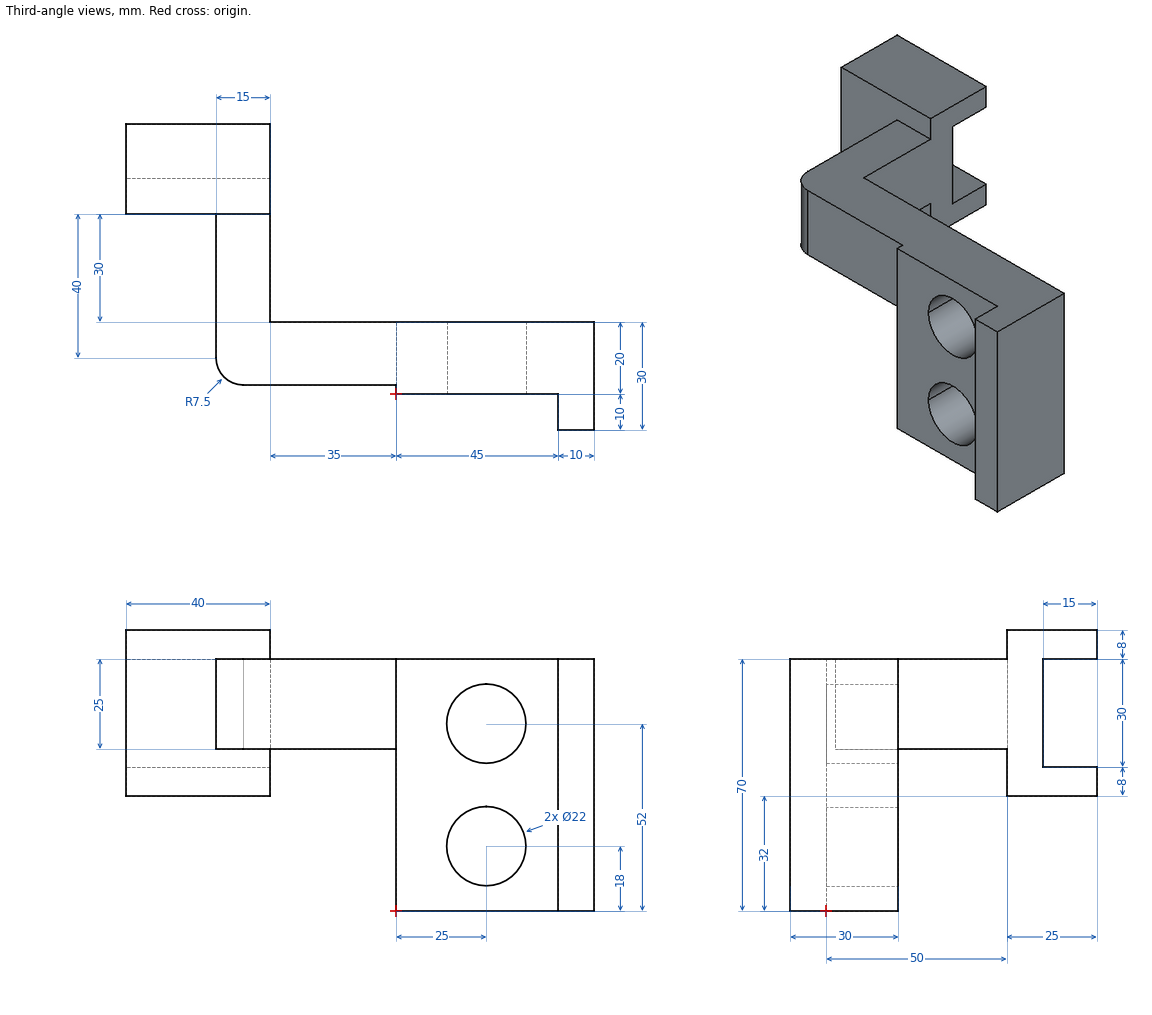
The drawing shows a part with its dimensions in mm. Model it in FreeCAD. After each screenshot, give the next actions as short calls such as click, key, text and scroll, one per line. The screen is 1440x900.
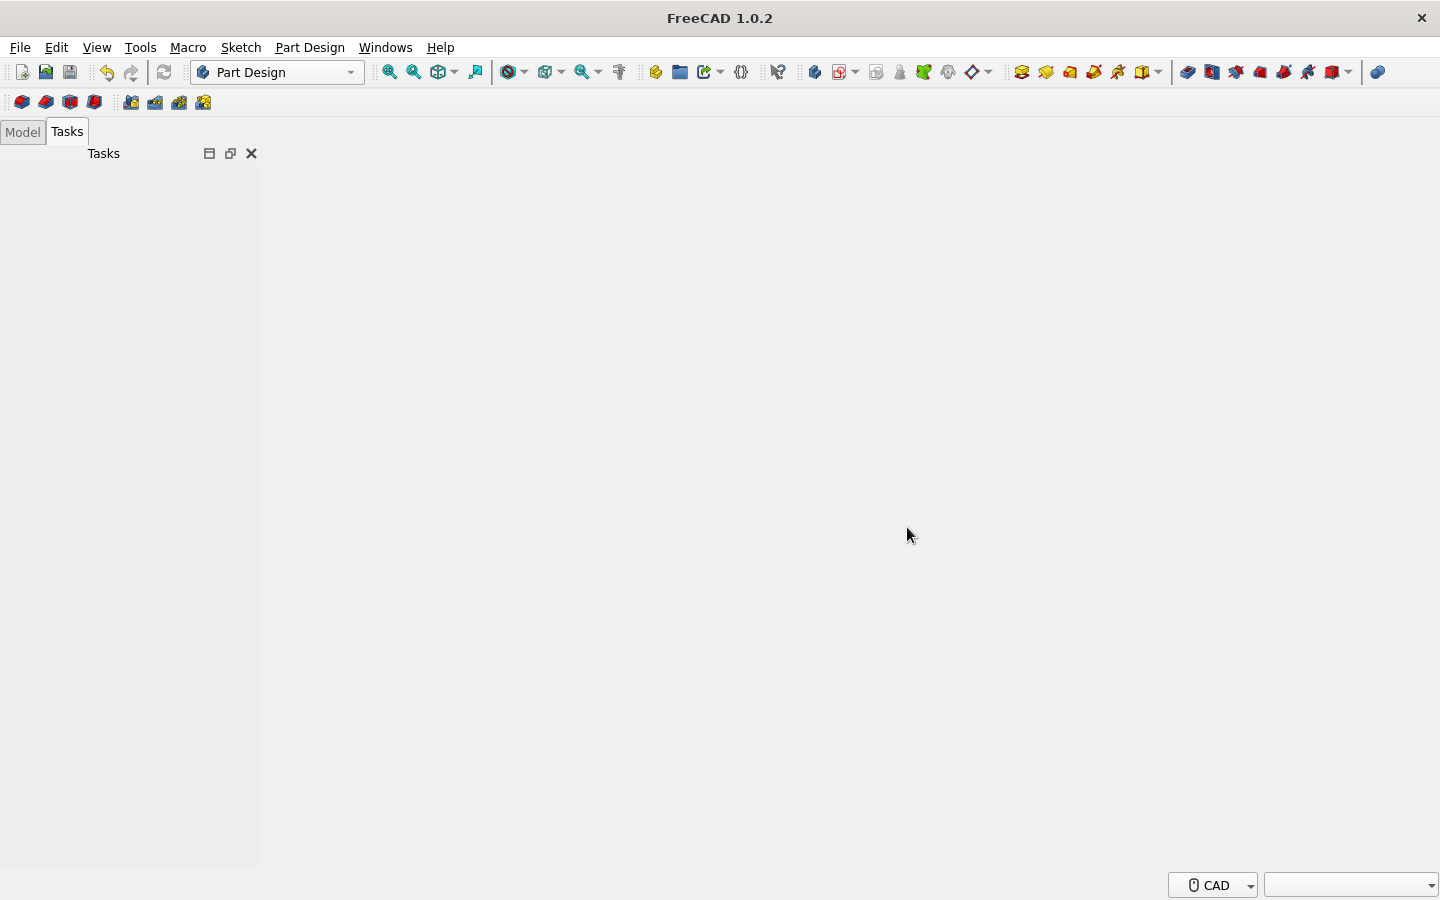
click(22, 72)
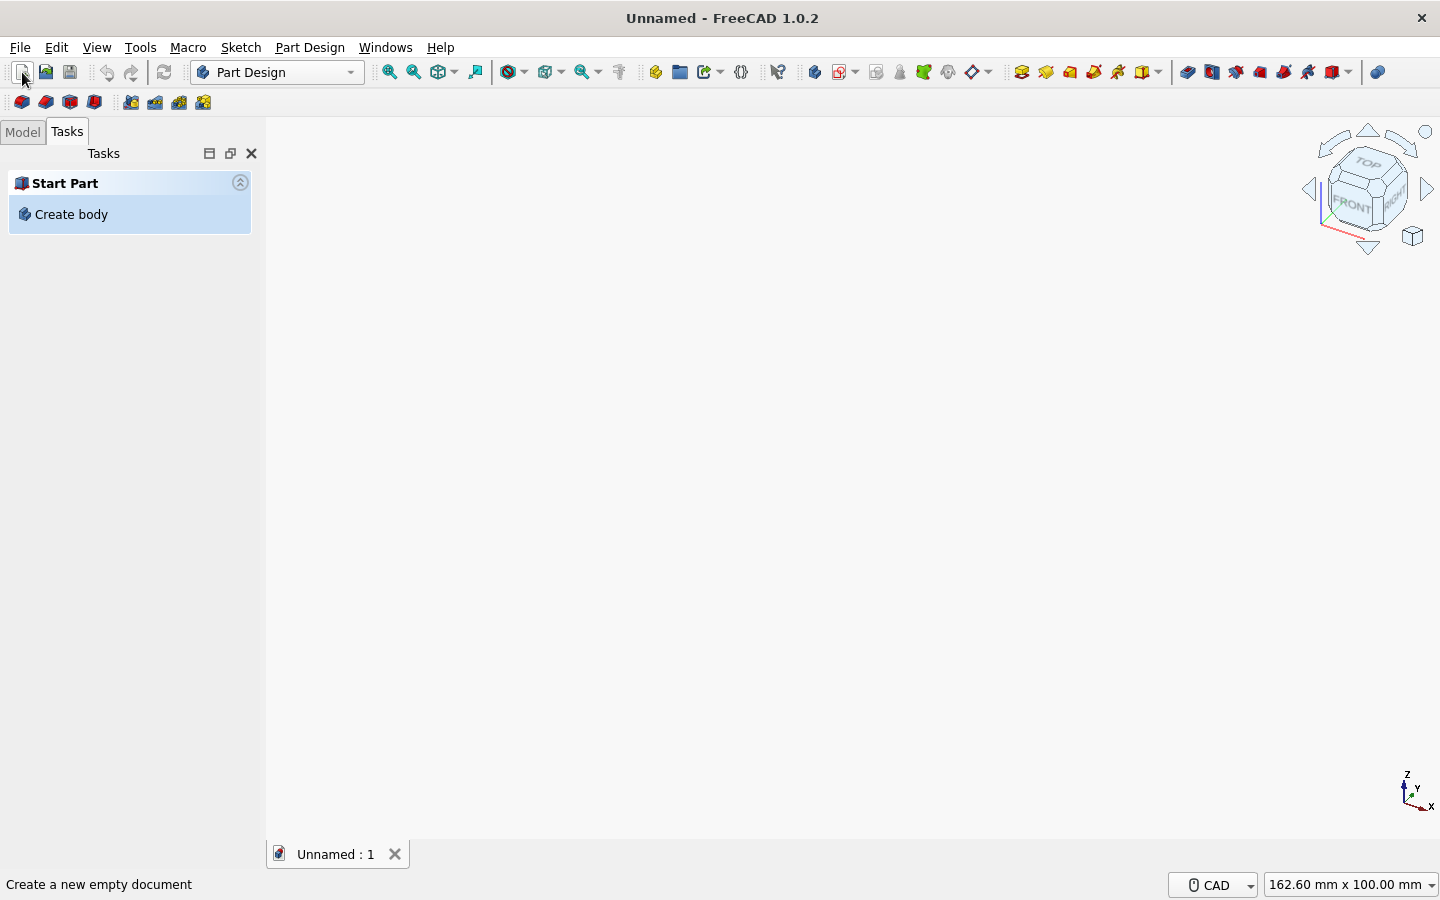
click(840, 72)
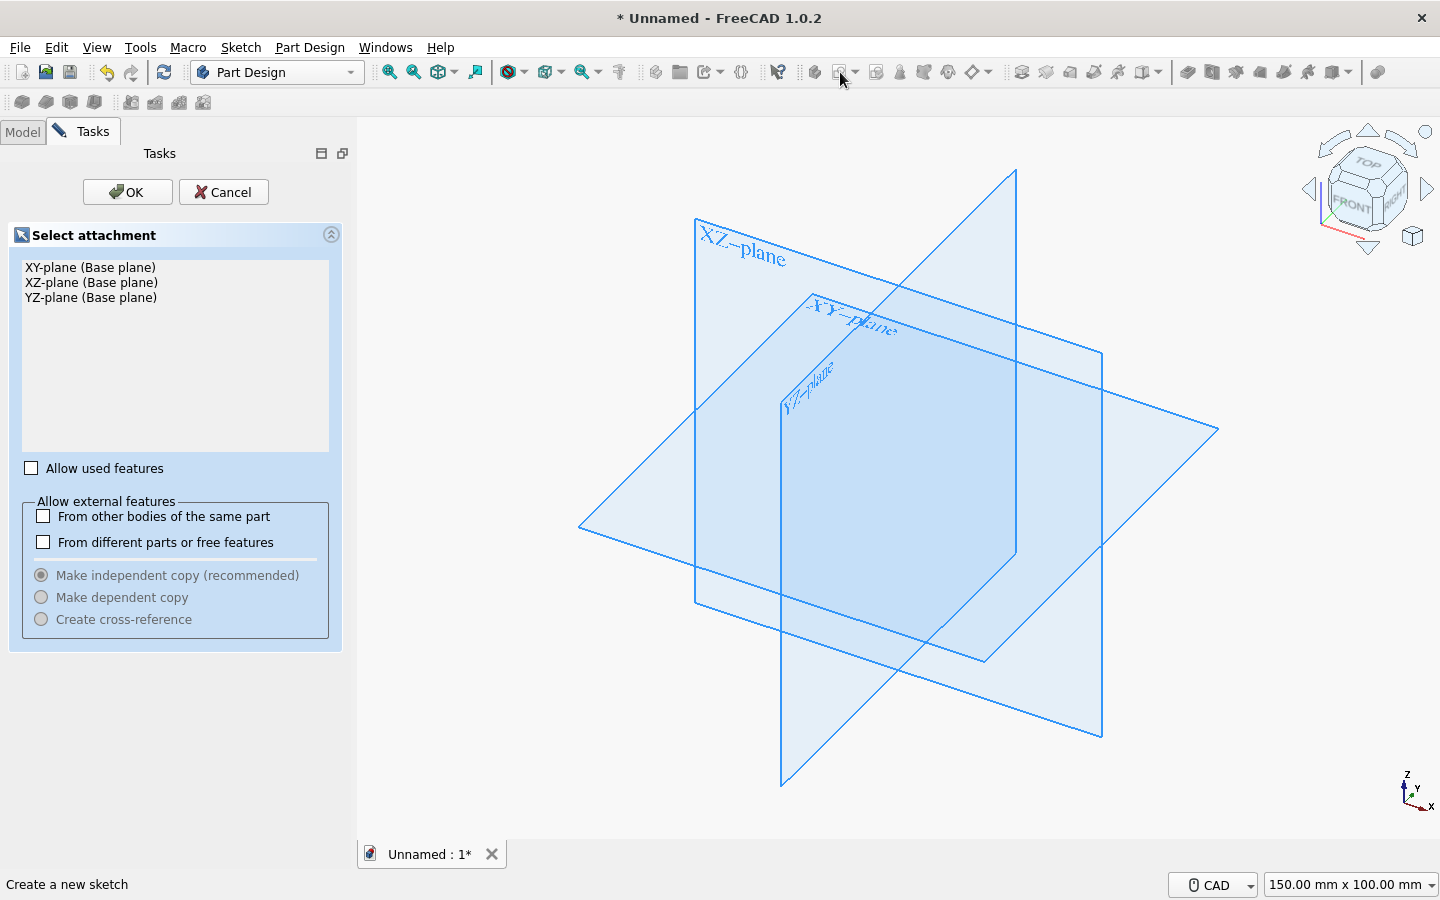
click(82, 268)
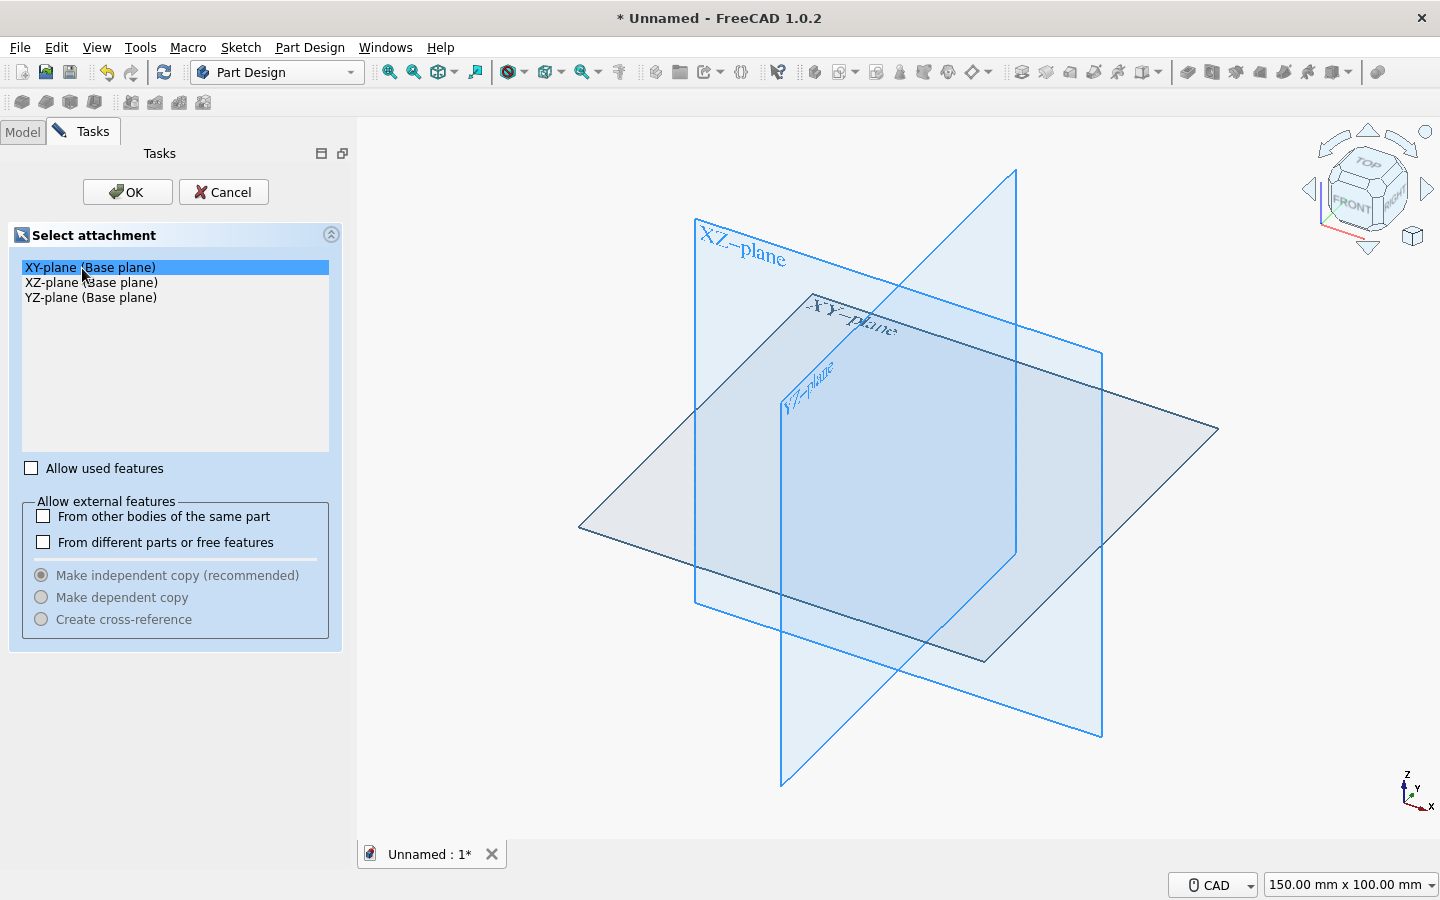
click(128, 192)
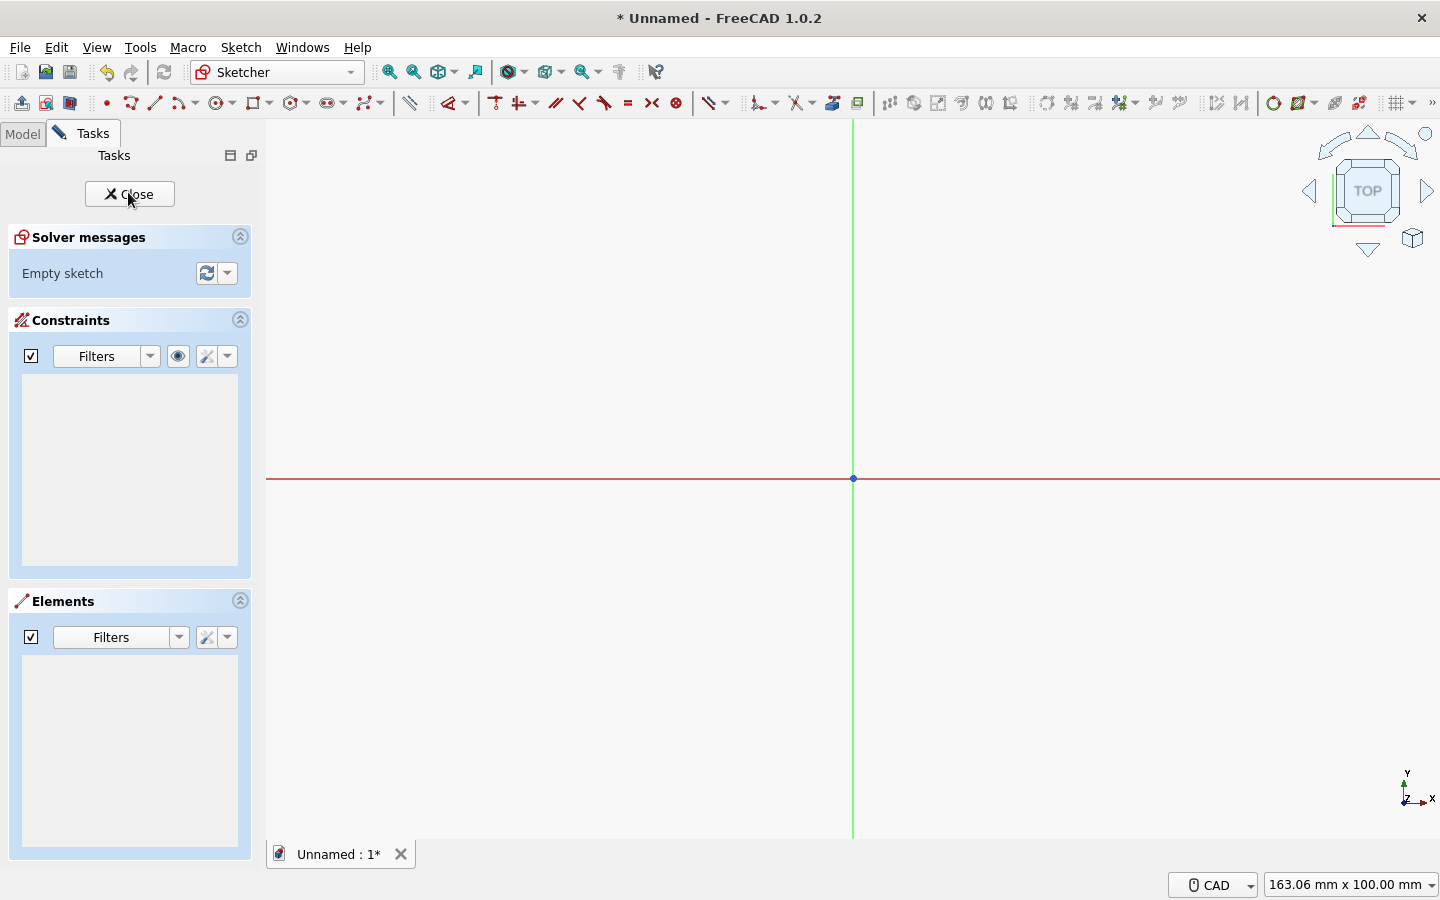
scroll(1275, 399, up, 3)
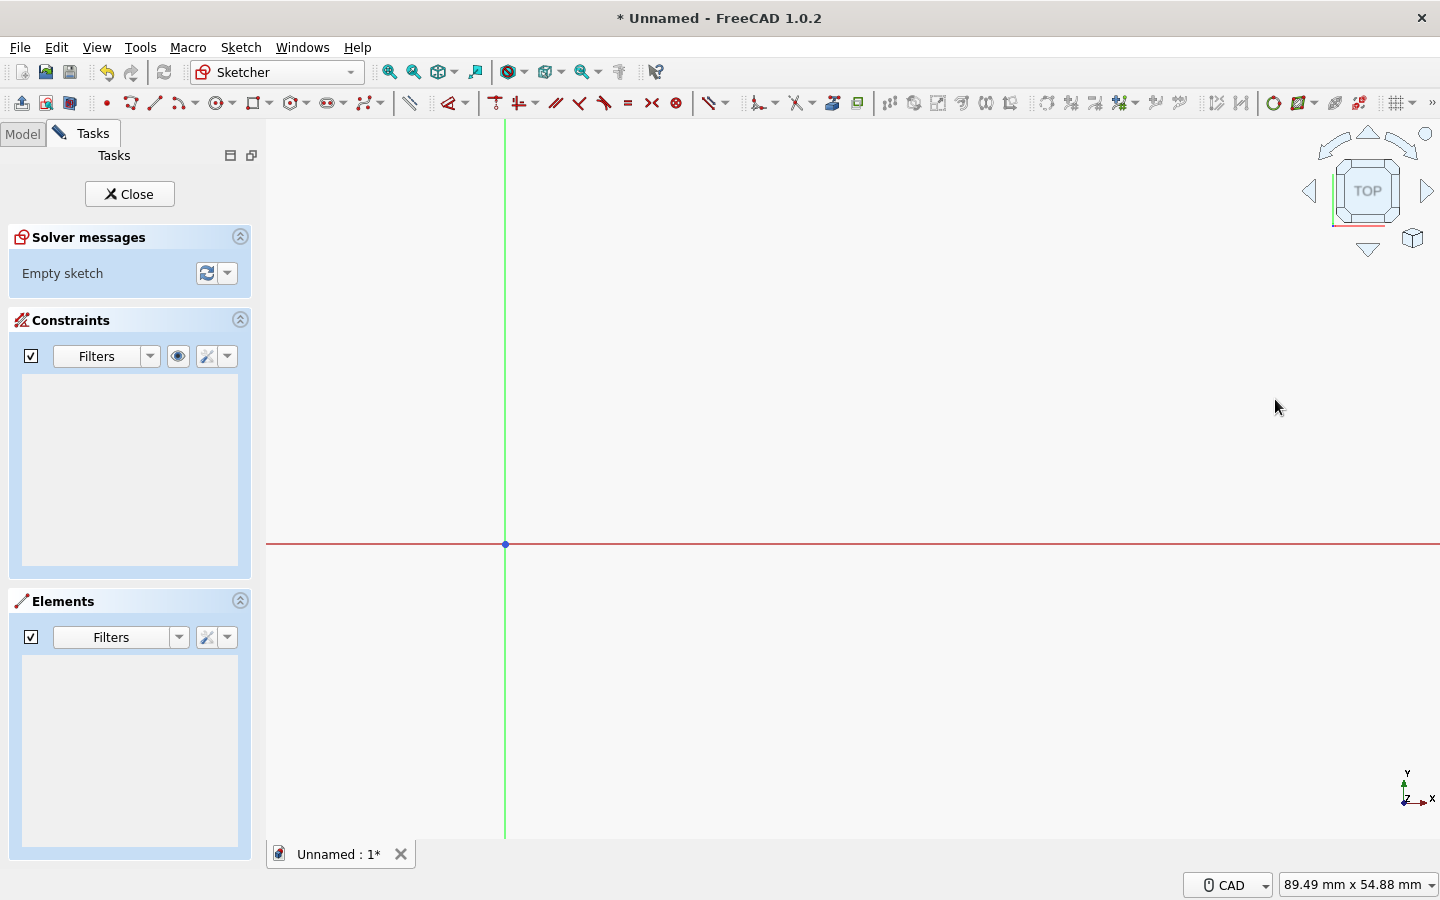
click(132, 104)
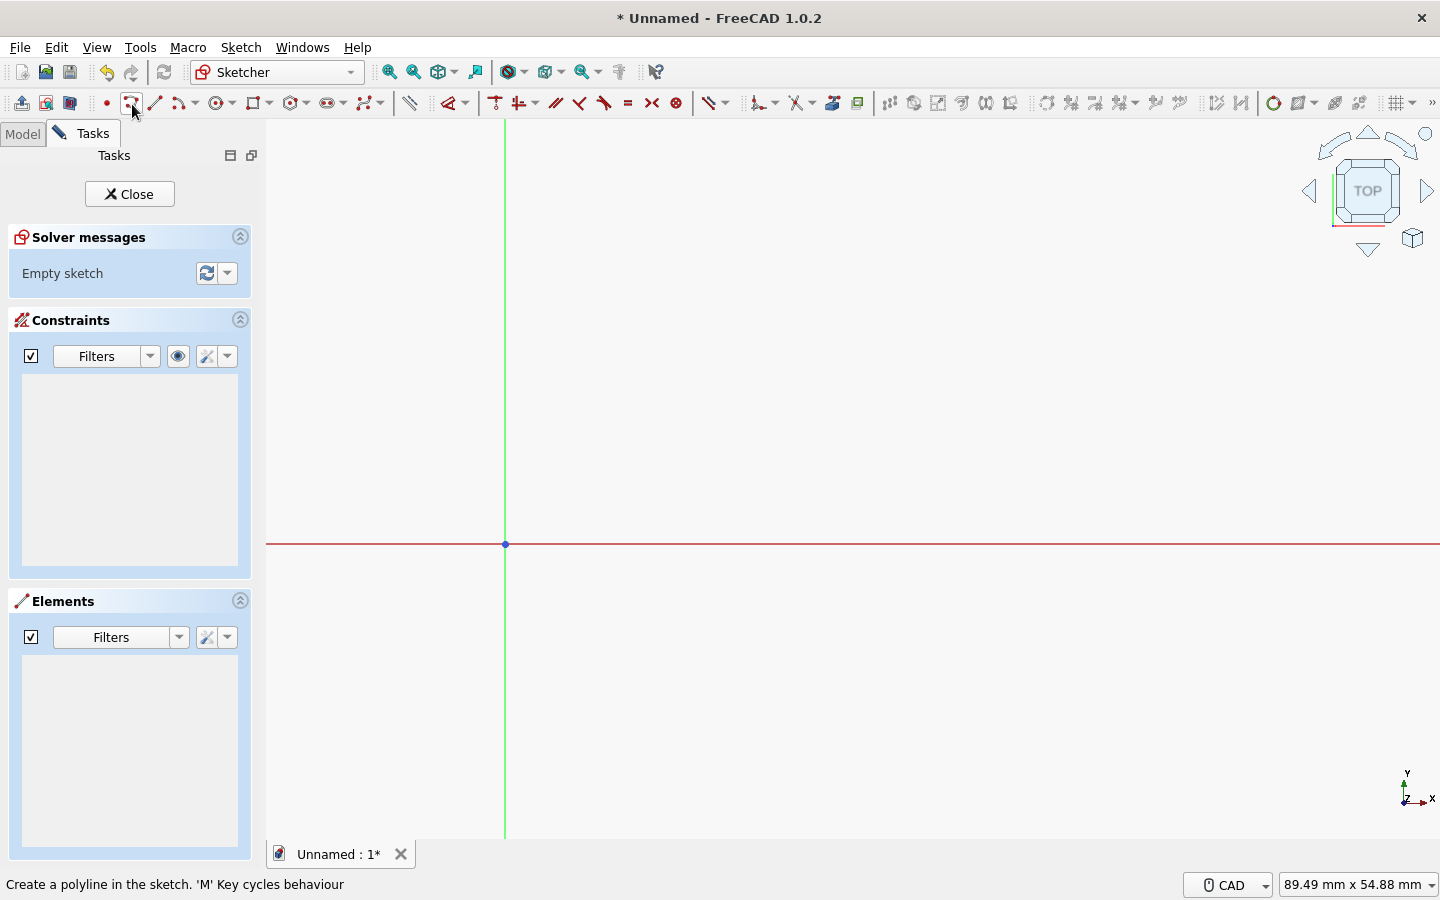
click(505, 544)
click(1096, 535)
click(1096, 676)
click(1227, 676)
click(1227, 282)
click(514, 282)
click(505, 544)
key(Escape)
key(Escape)